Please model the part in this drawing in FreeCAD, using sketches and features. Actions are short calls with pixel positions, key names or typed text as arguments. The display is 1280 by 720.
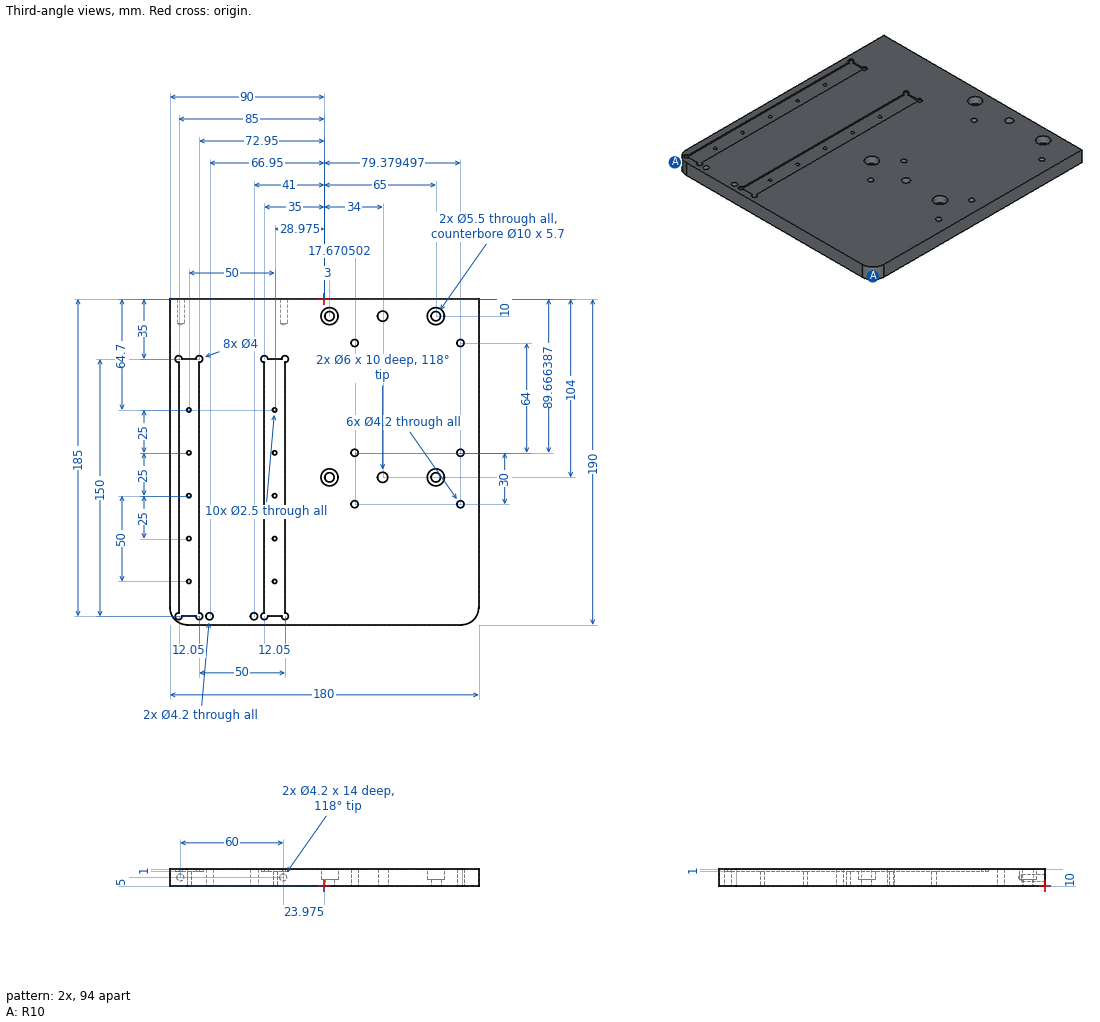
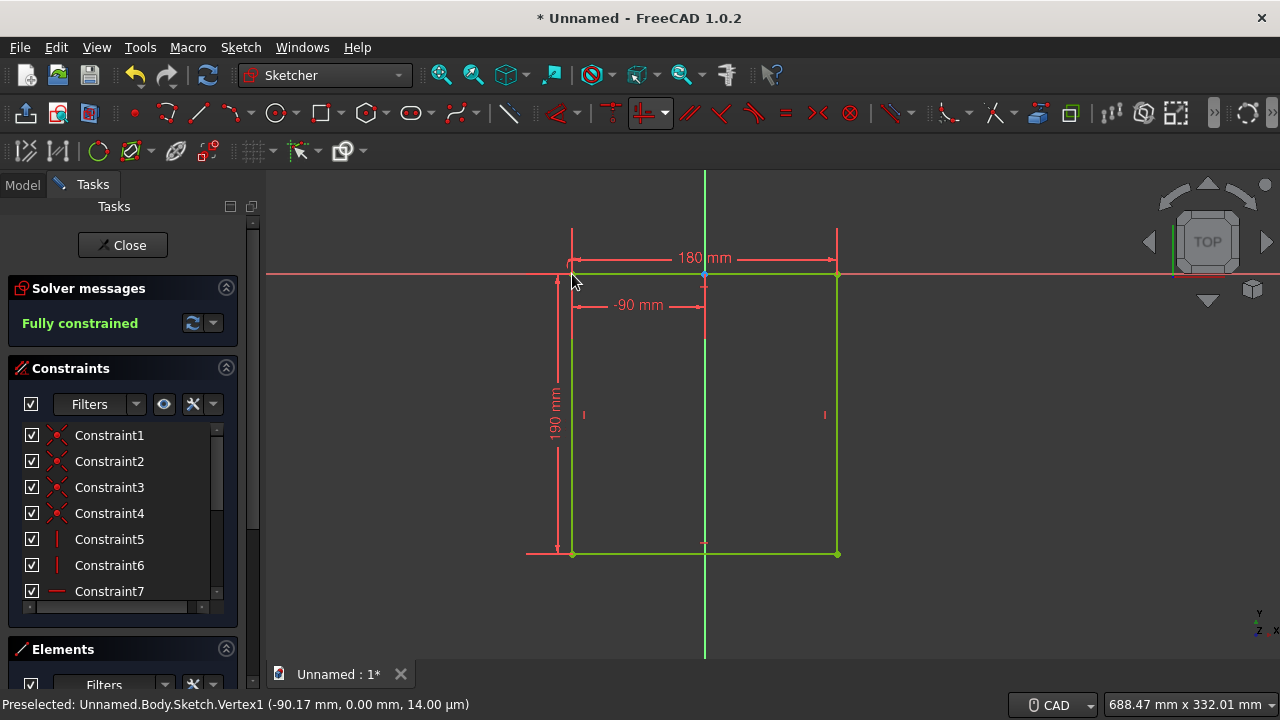
click(123, 245)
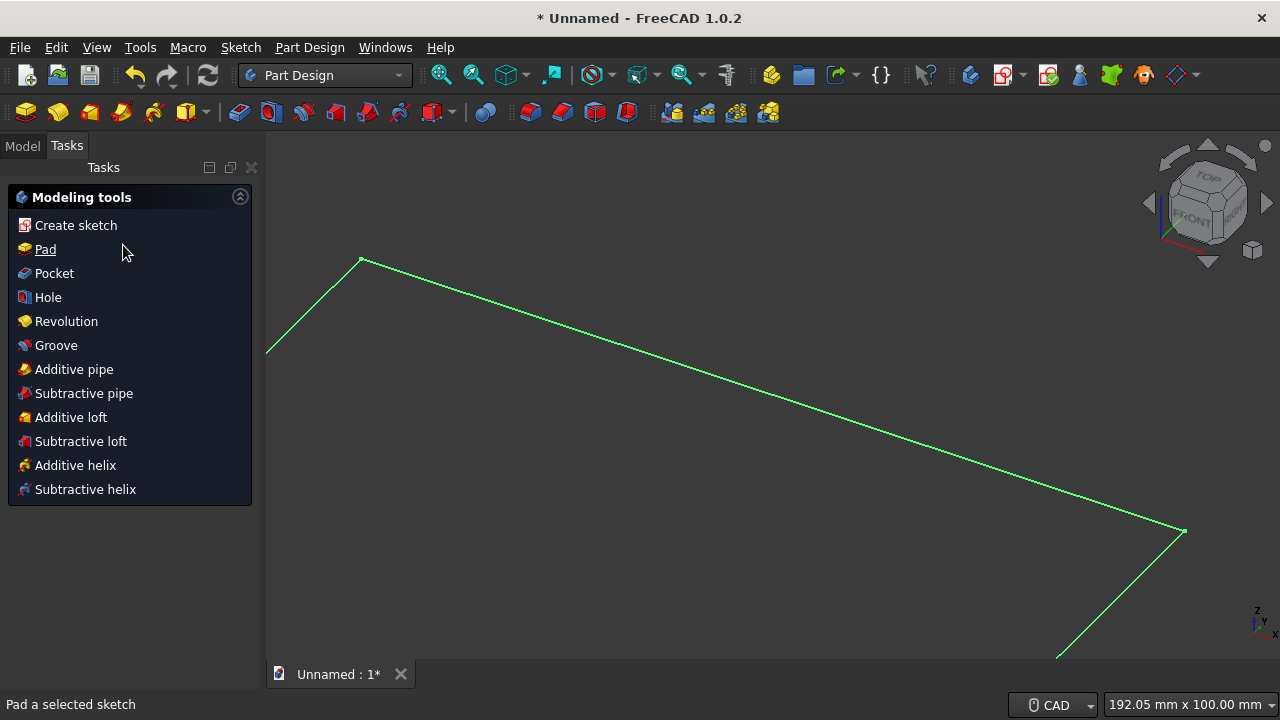
click(26, 112)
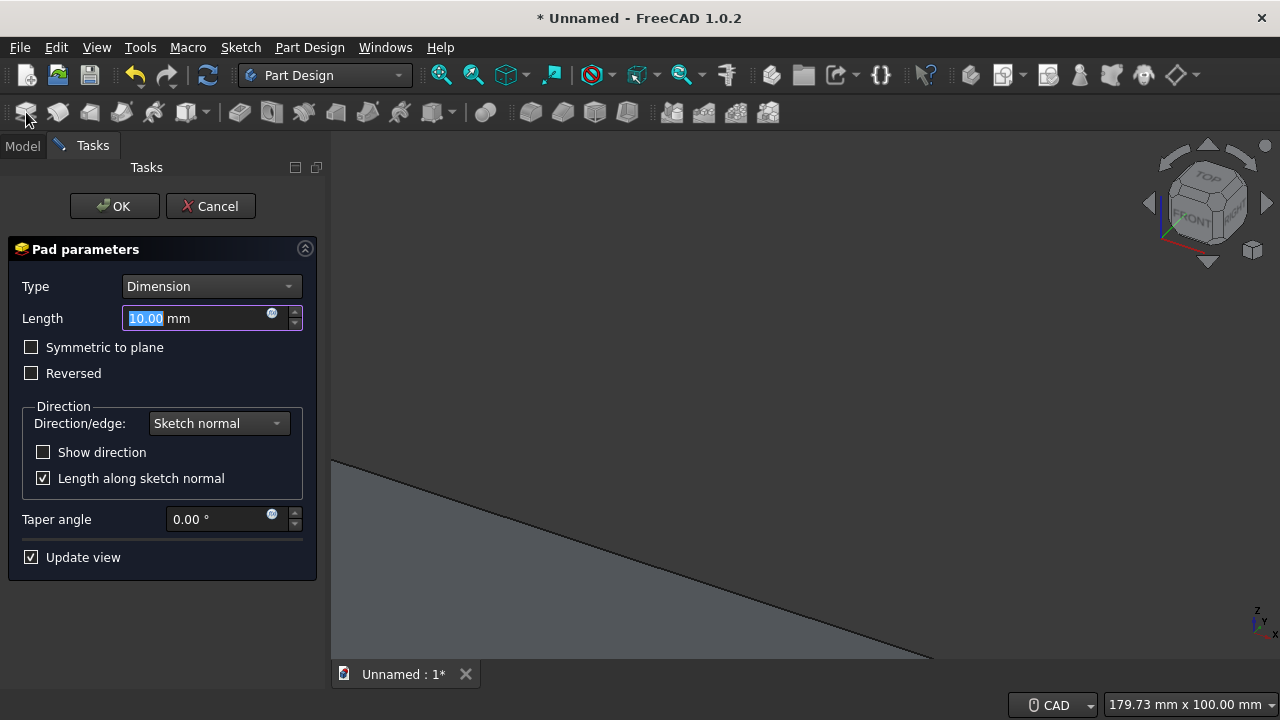
text(10)
key(Tab)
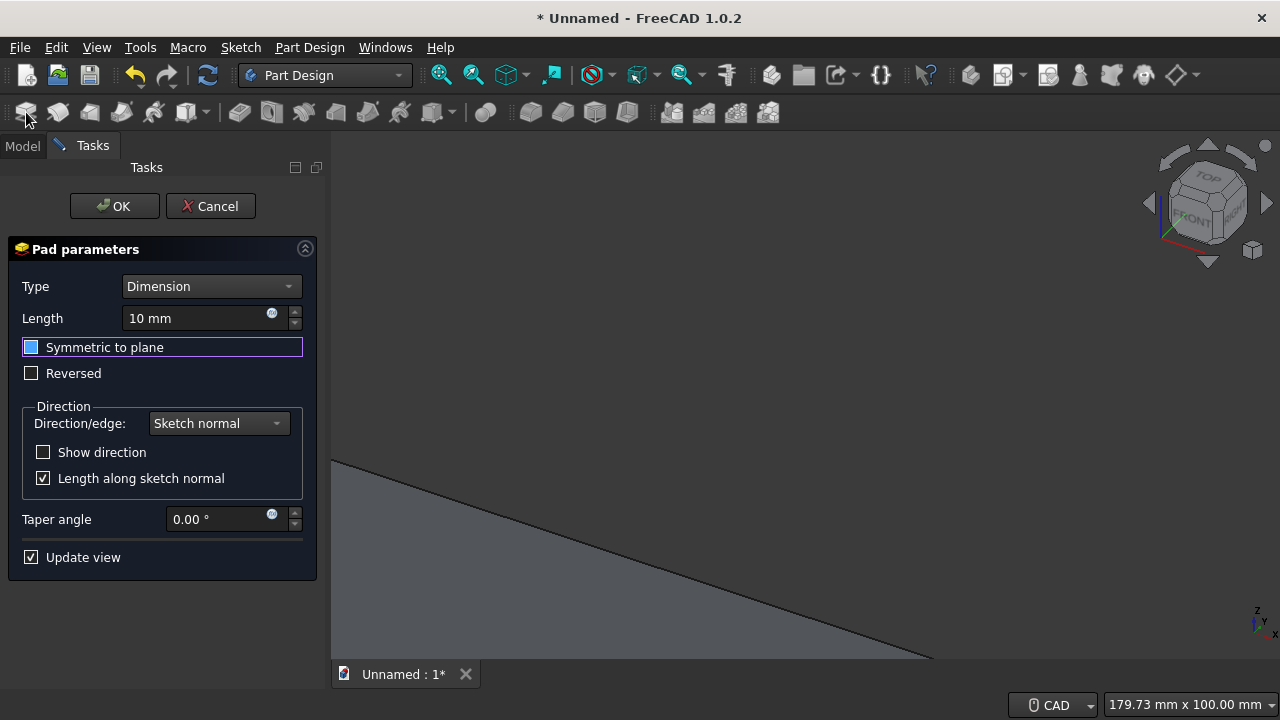
click(115, 206)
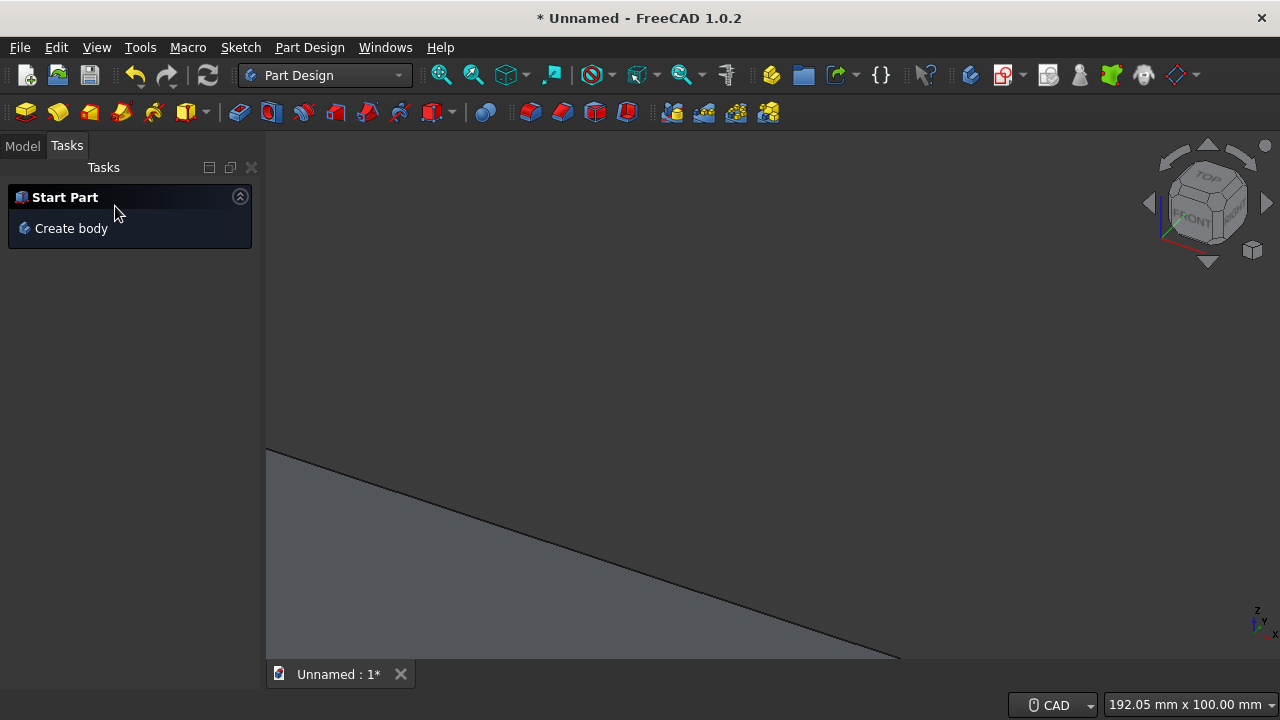
click(442, 76)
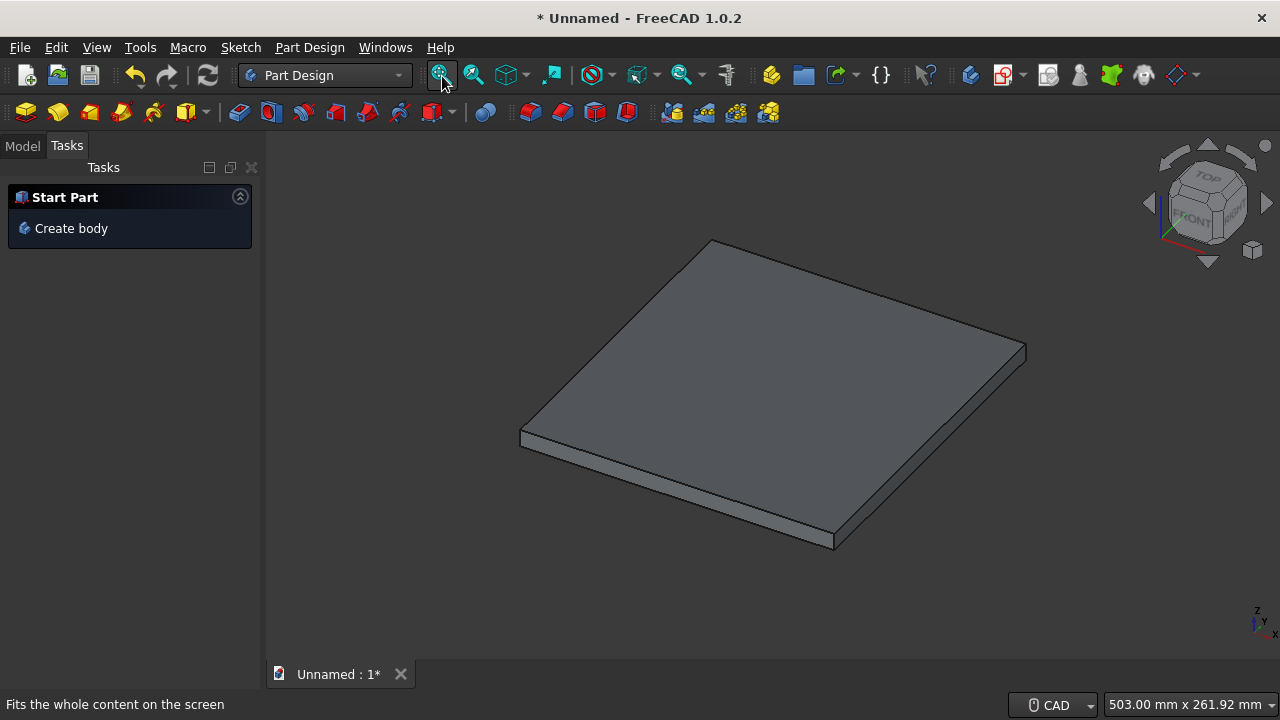
click(773, 386)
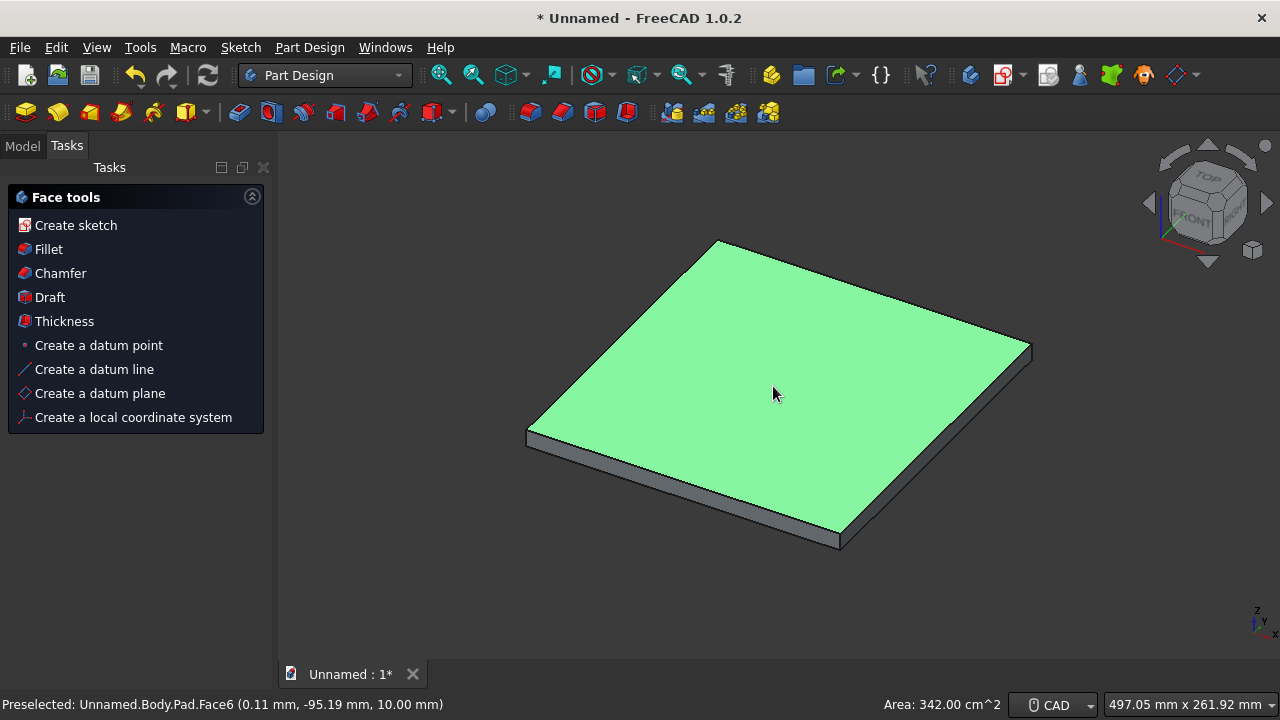
click(1004, 76)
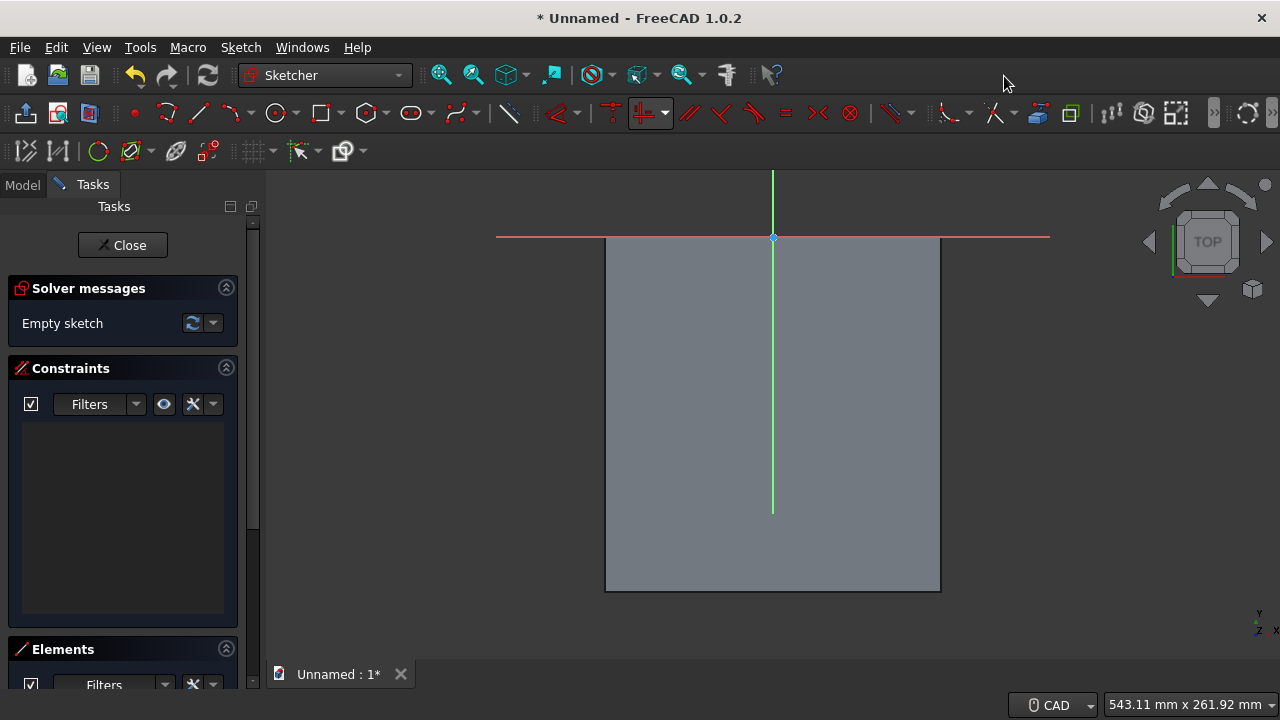
scroll(870, 207, up, 8)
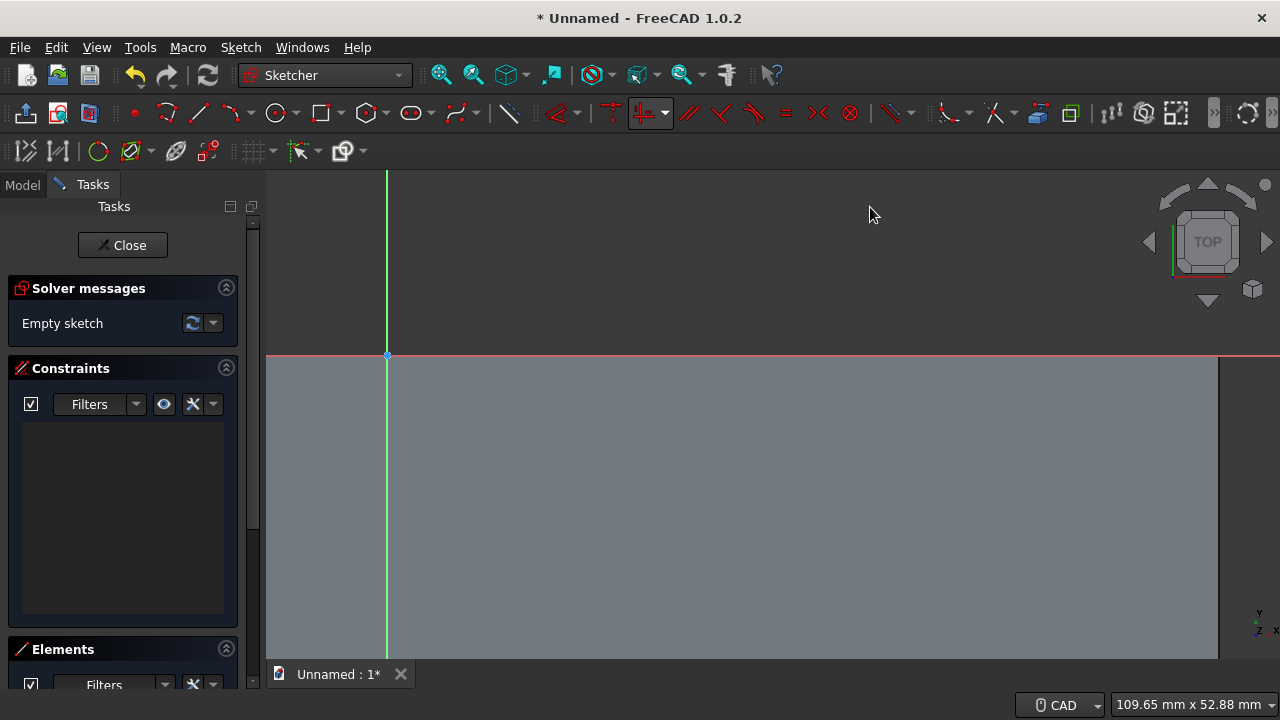
key(g)
key(c)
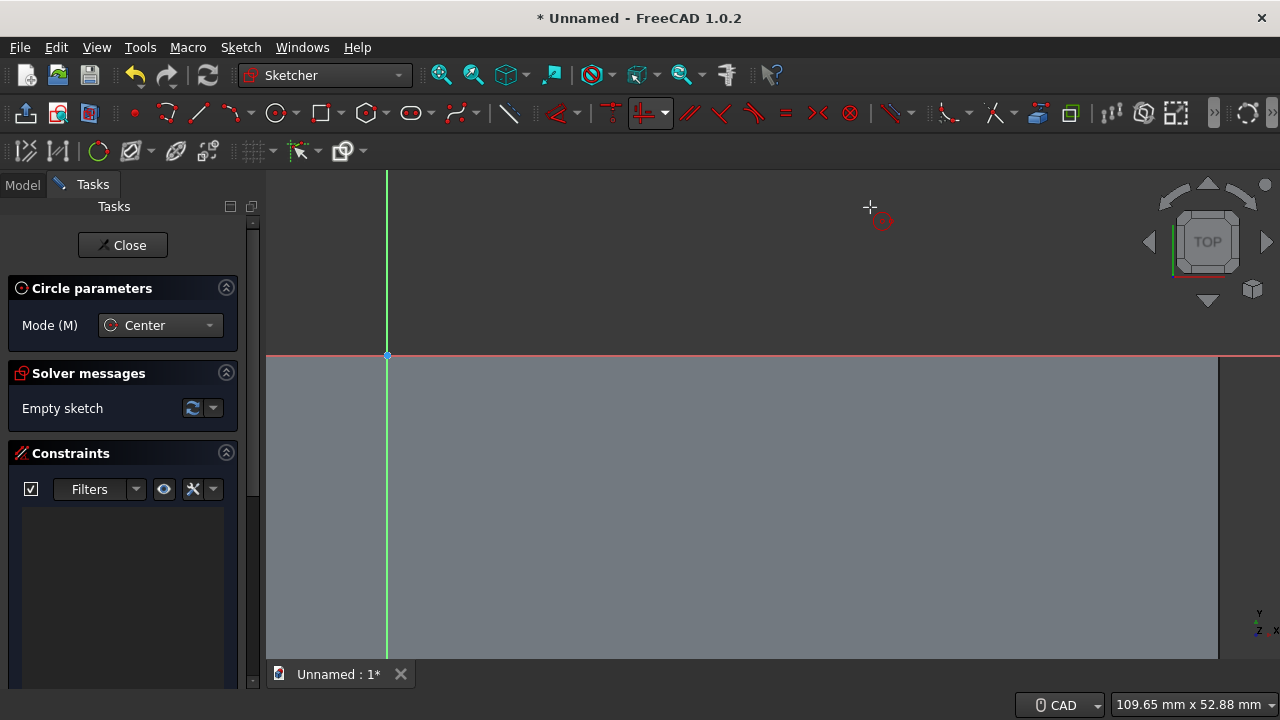
click(988, 448)
move(1006, 430)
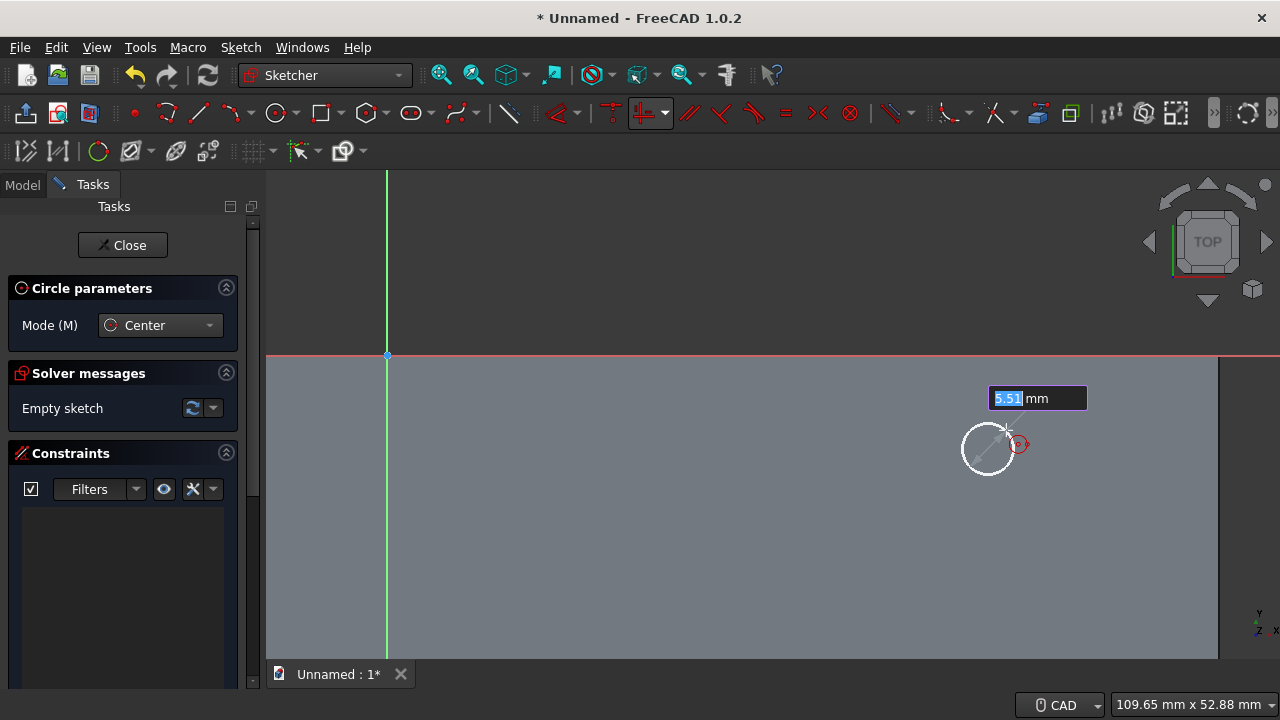
text(5.5)
key(Return)